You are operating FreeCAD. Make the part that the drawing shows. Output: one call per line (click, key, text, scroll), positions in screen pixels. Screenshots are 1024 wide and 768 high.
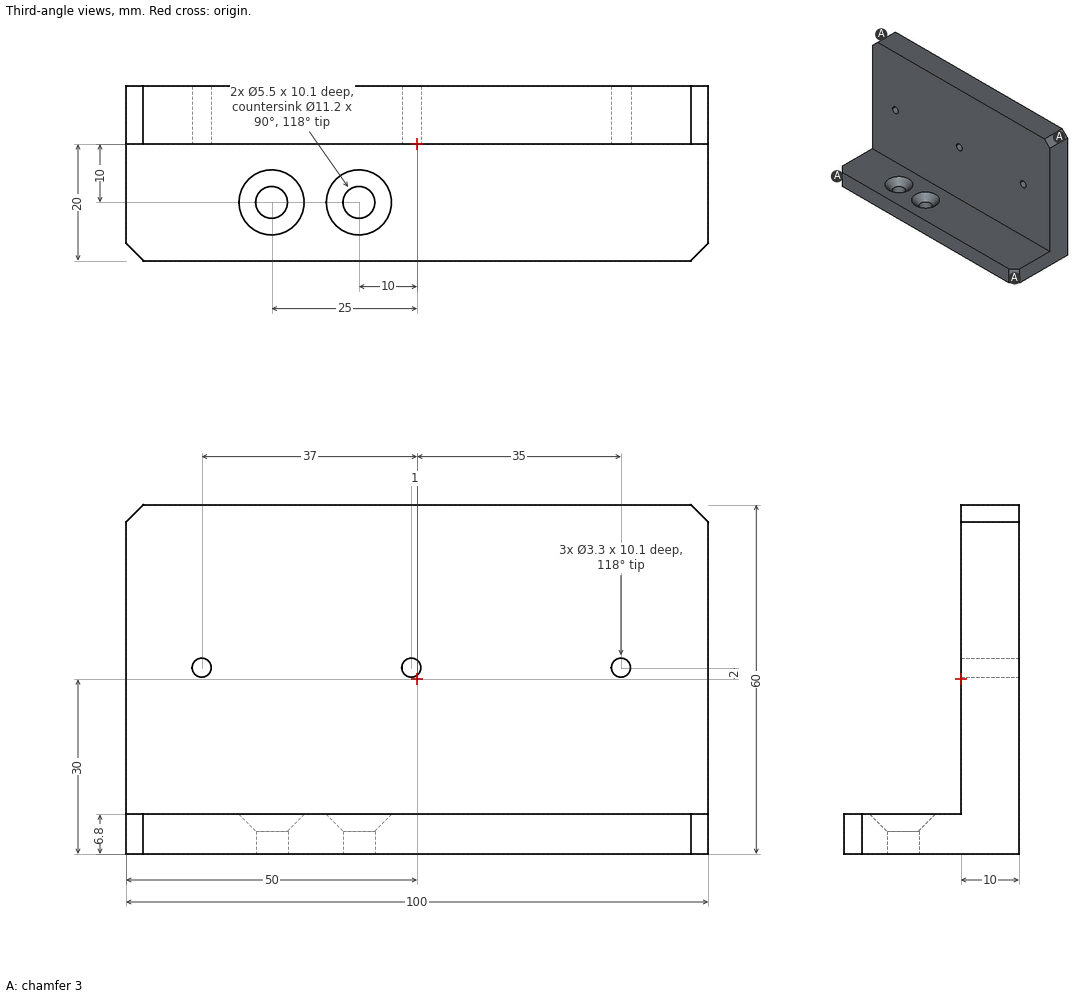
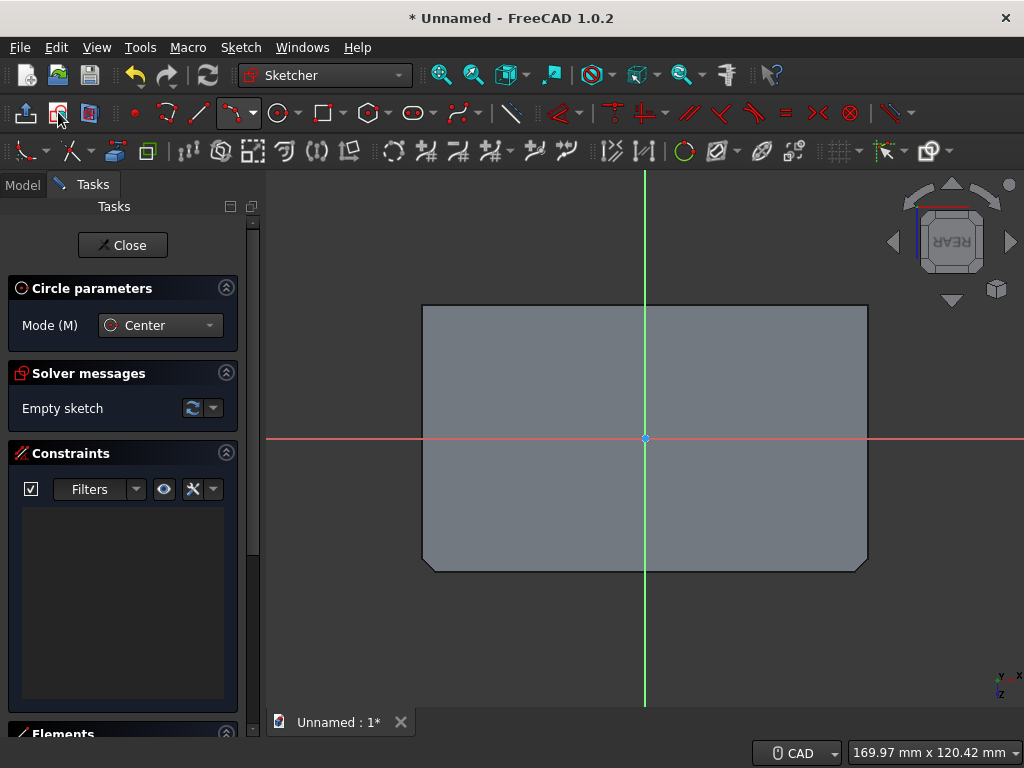
scroll(801, 447, up, 6)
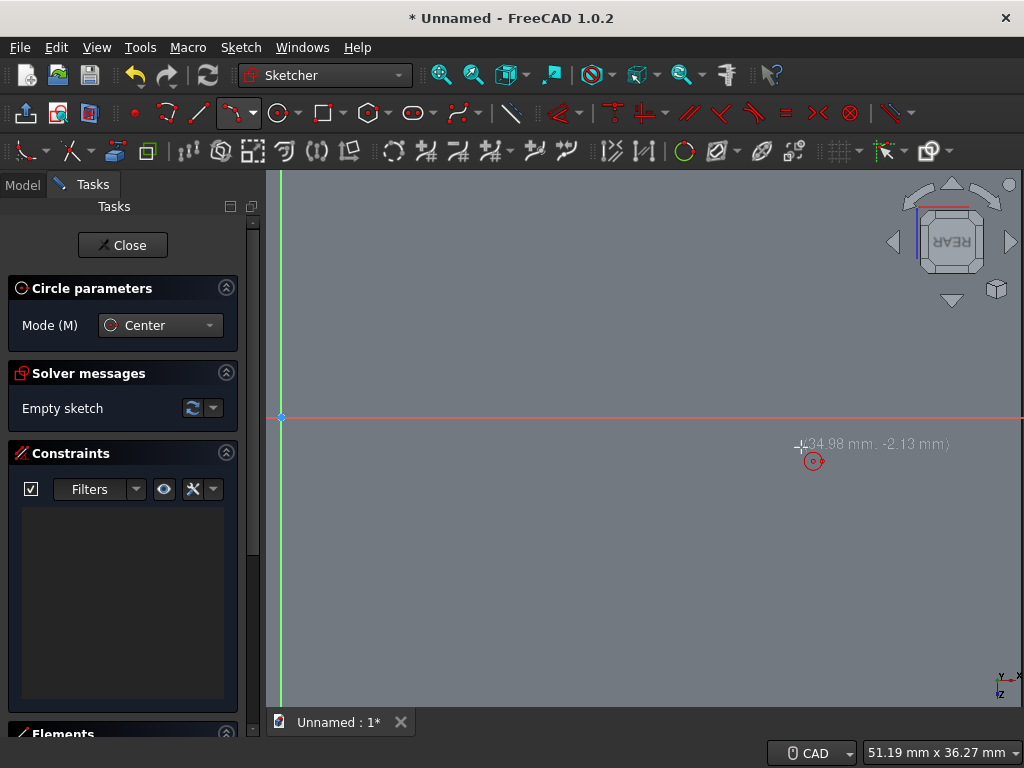
click(800, 447)
click(817, 464)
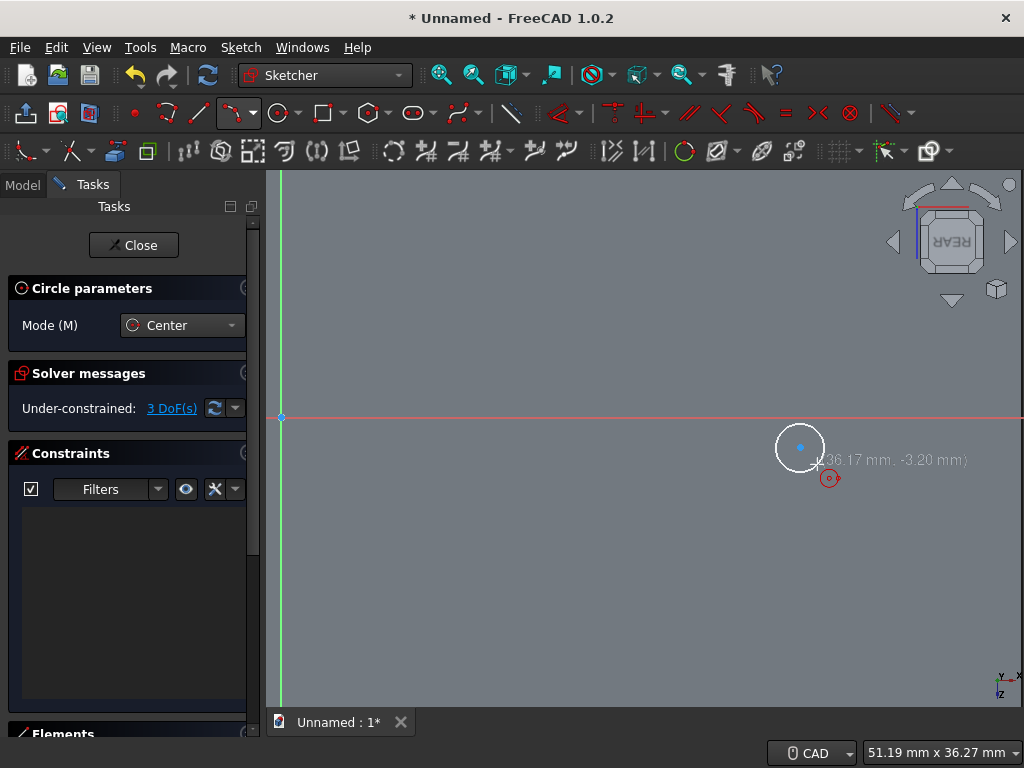
scroll(757, 435, down, 5)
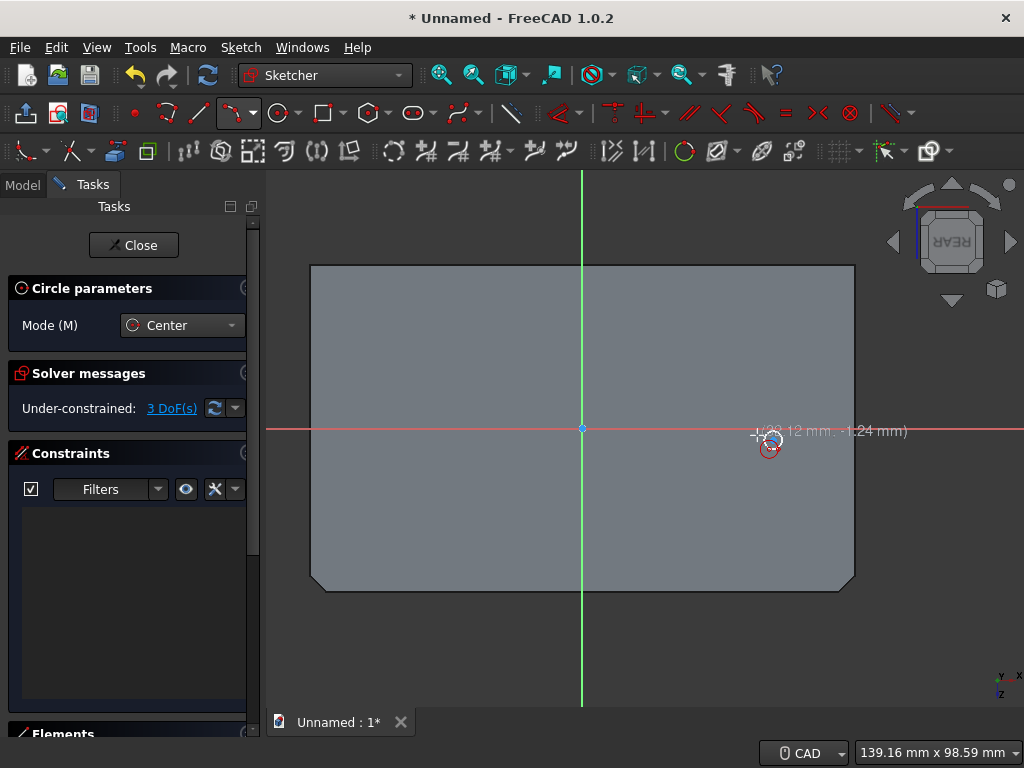
scroll(381, 440, up, 5)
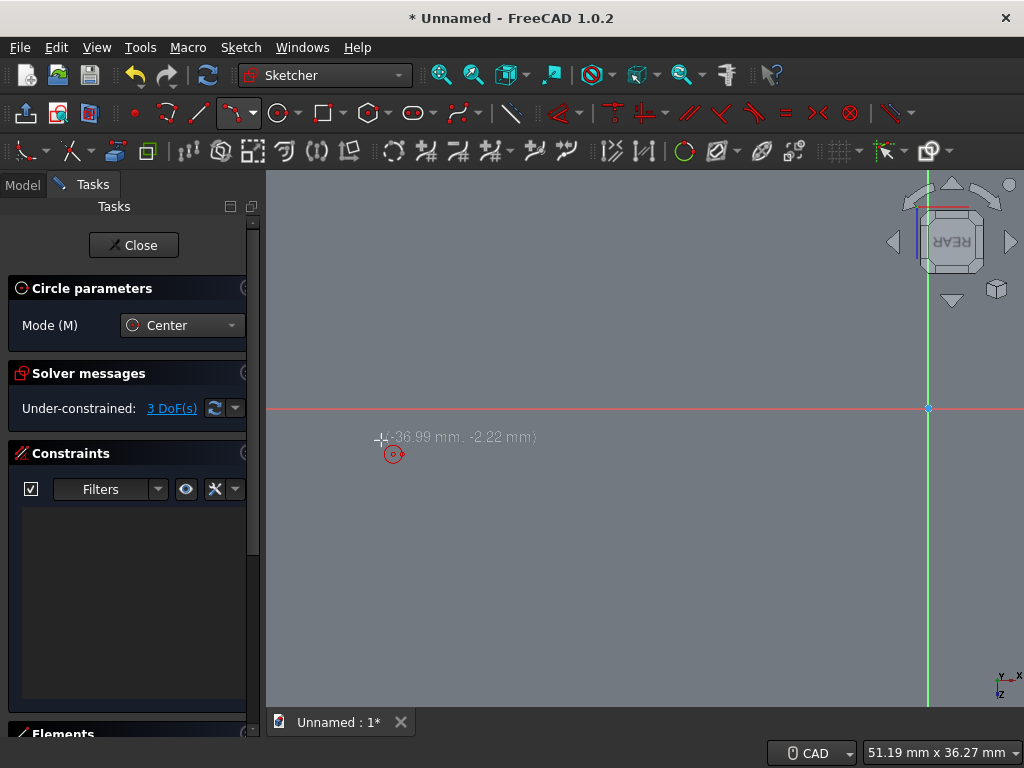
click(381, 439)
click(398, 456)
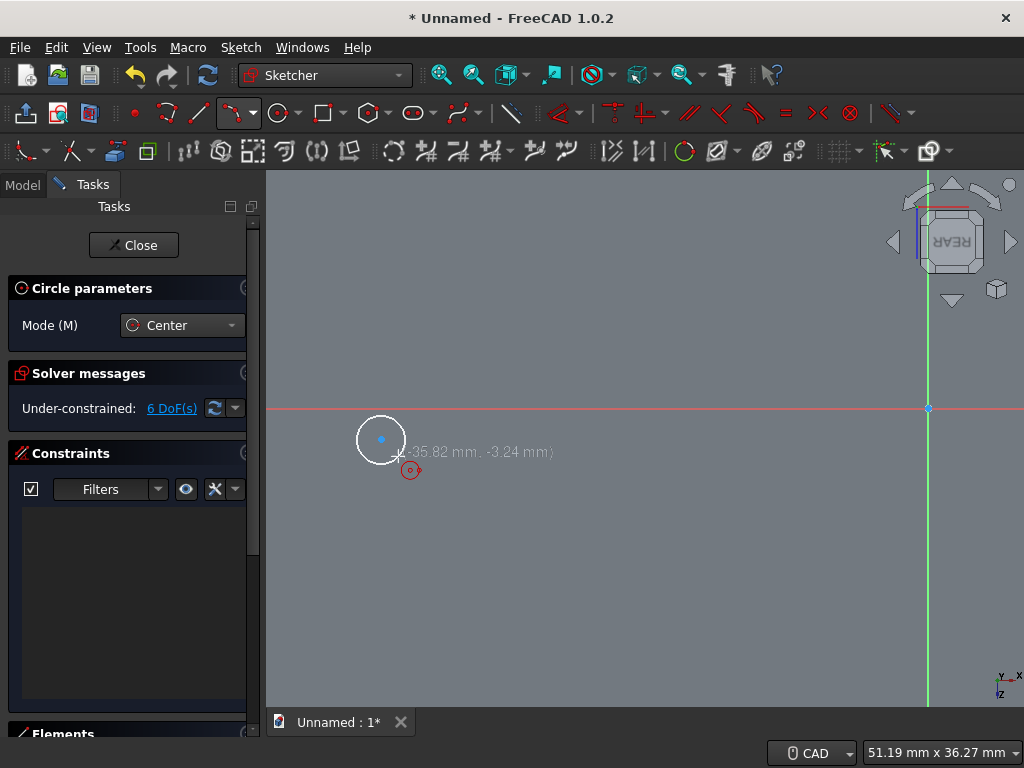
scroll(380, 440, down, 5)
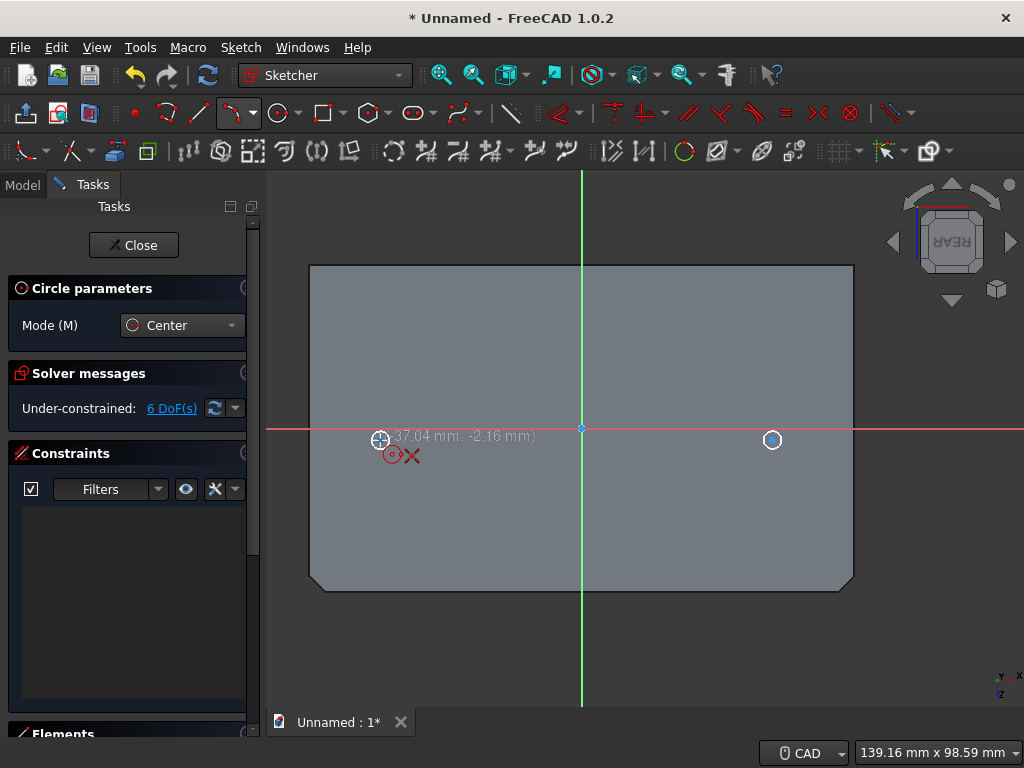
scroll(576, 440, up, 6)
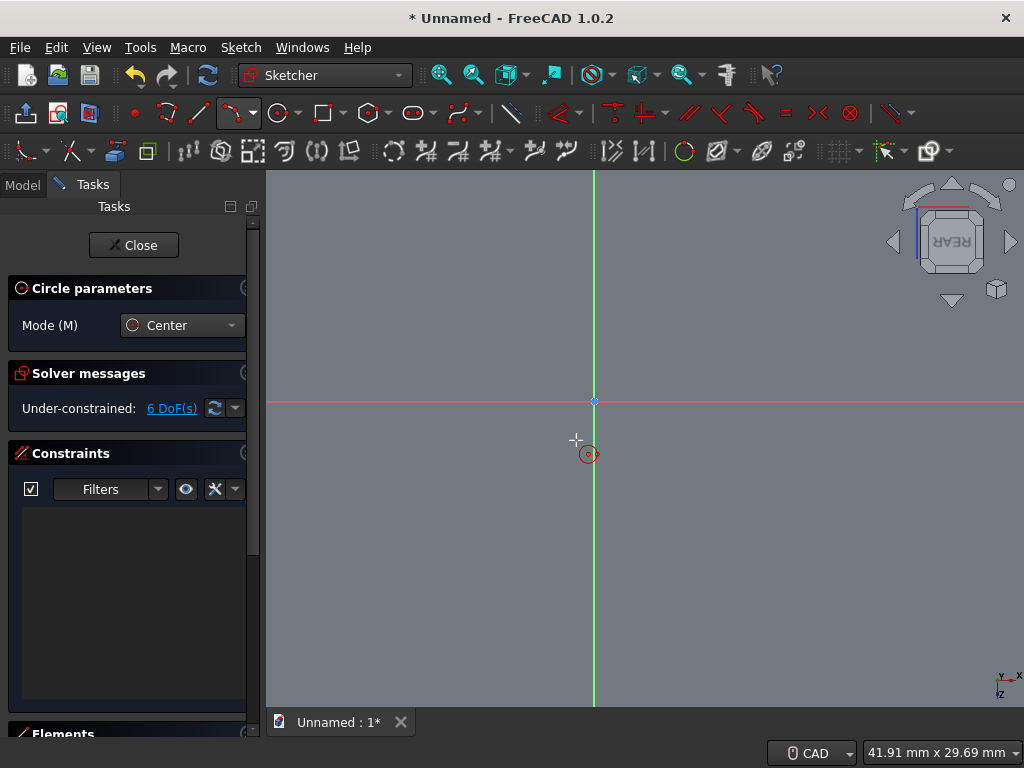
click(576, 438)
click(555, 417)
key(Escape)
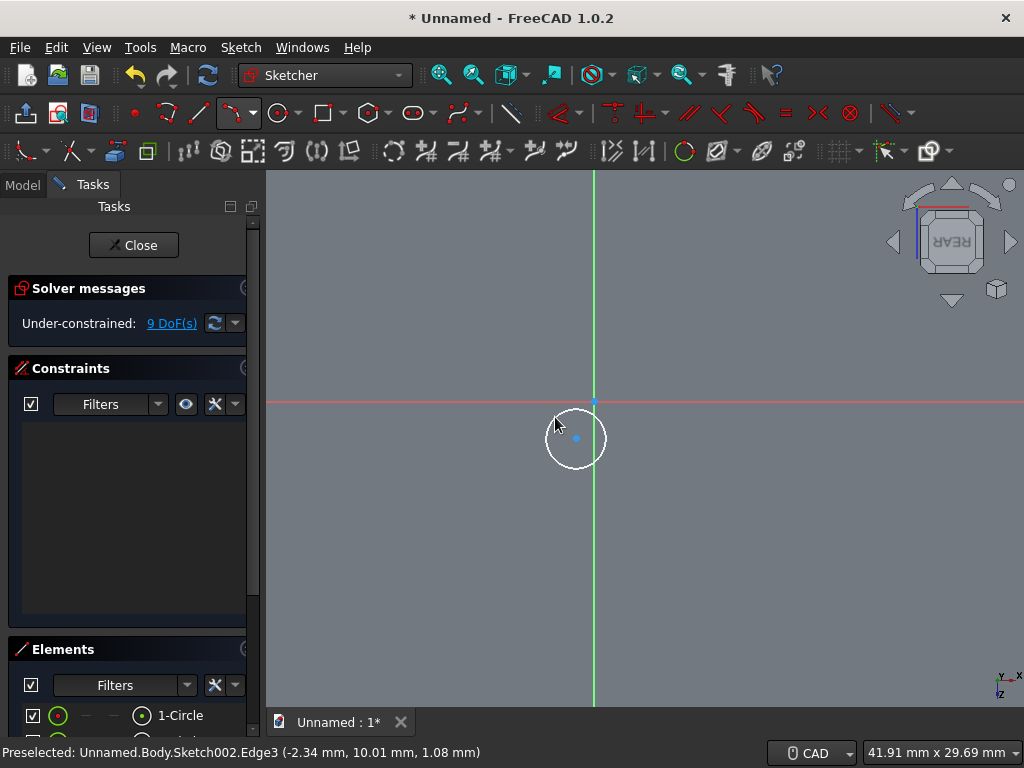
scroll(577, 440, down, 6)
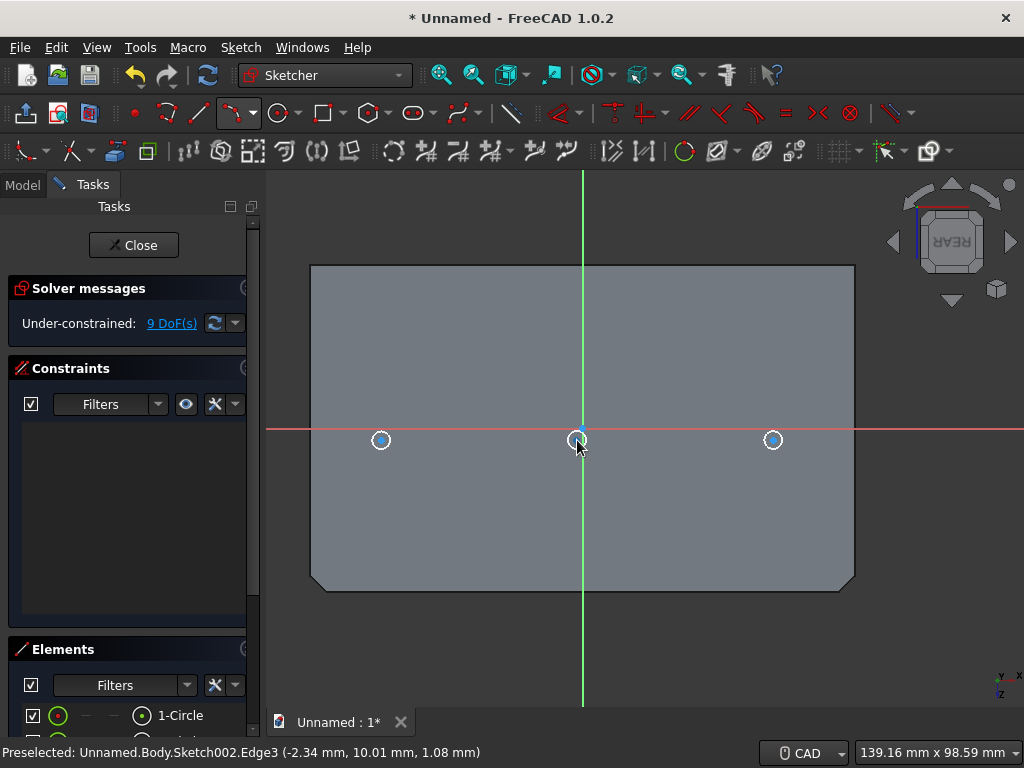
scroll(780, 434, up, 6)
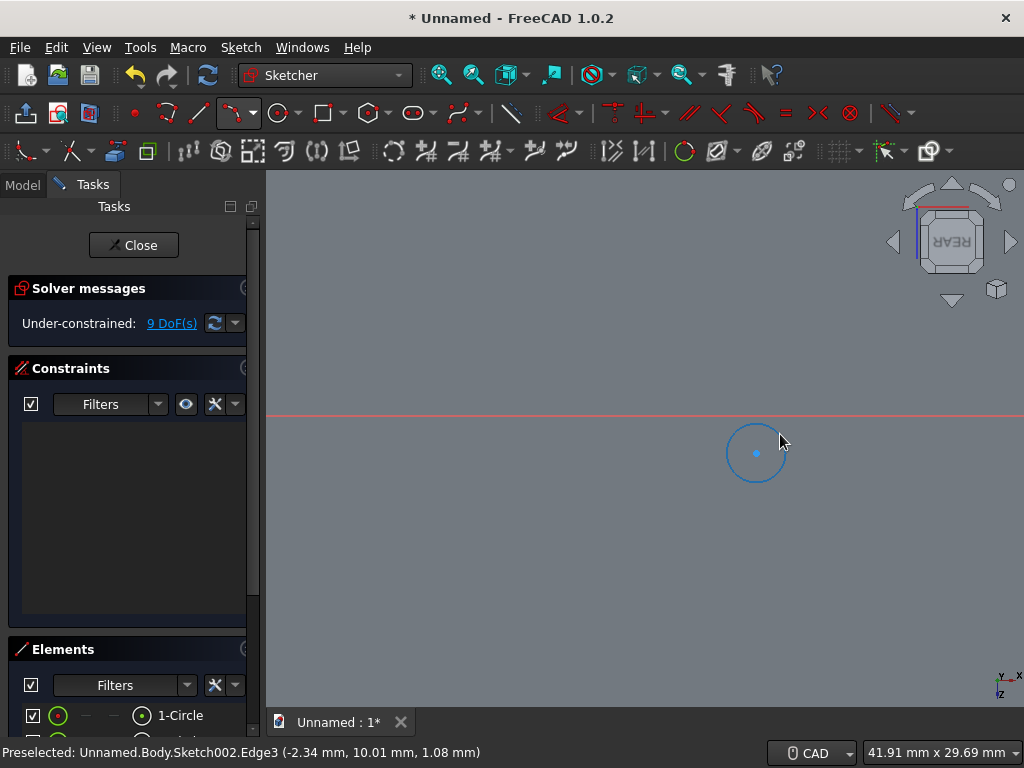
click(777, 432)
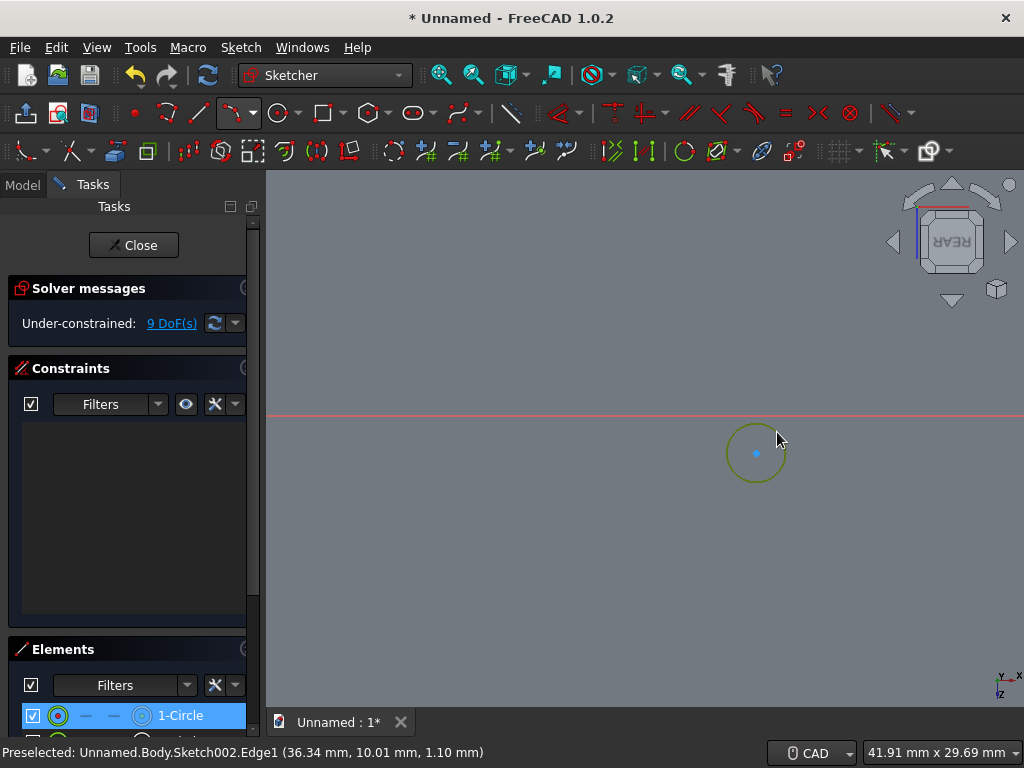
scroll(780, 434, down, 6)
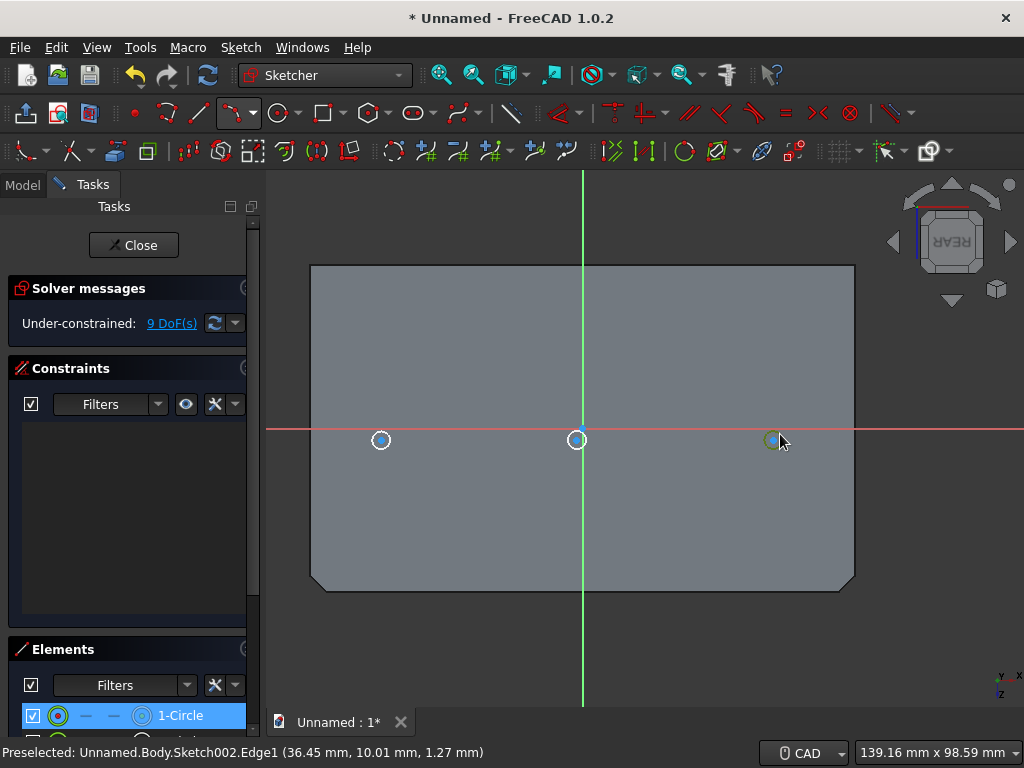
scroll(387, 434, up, 5)